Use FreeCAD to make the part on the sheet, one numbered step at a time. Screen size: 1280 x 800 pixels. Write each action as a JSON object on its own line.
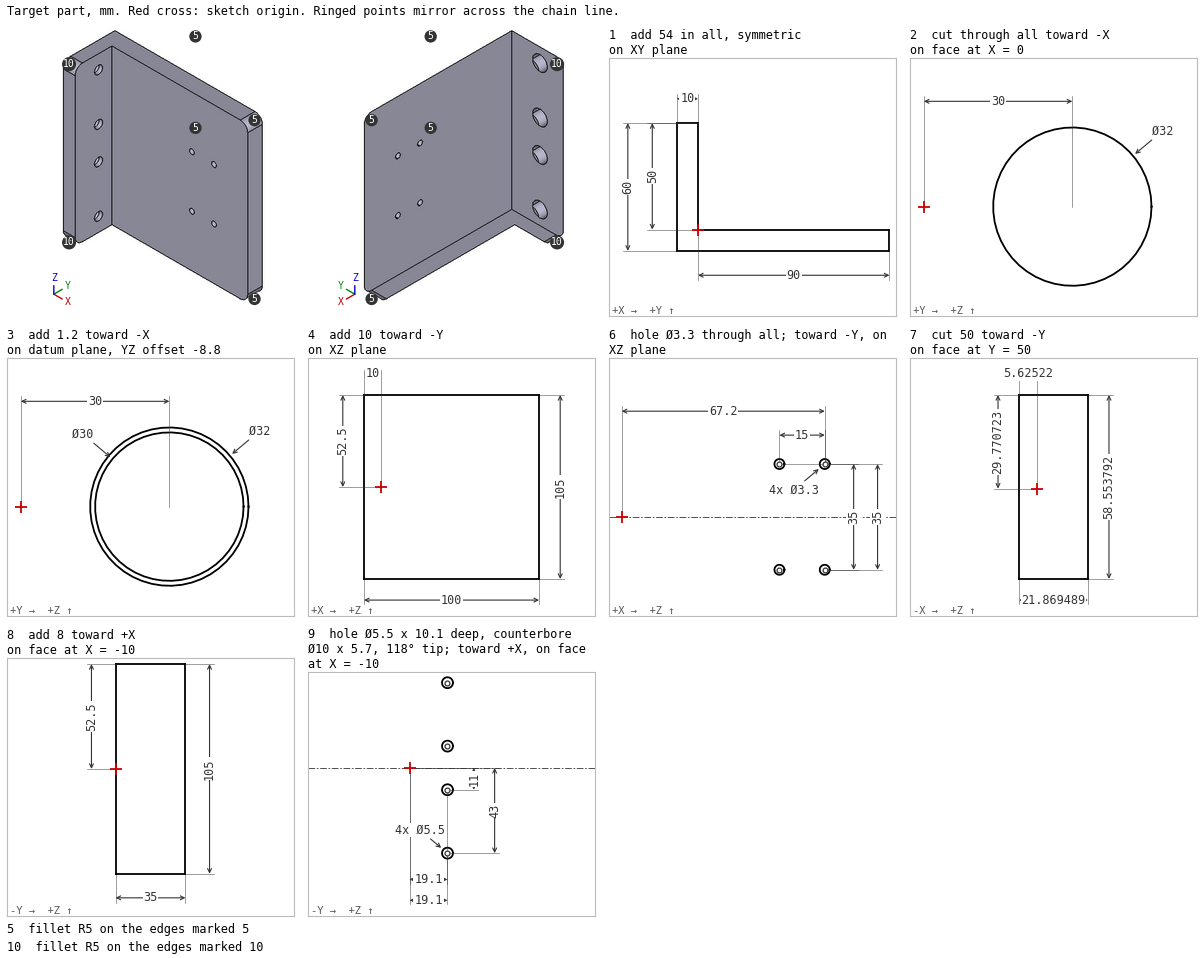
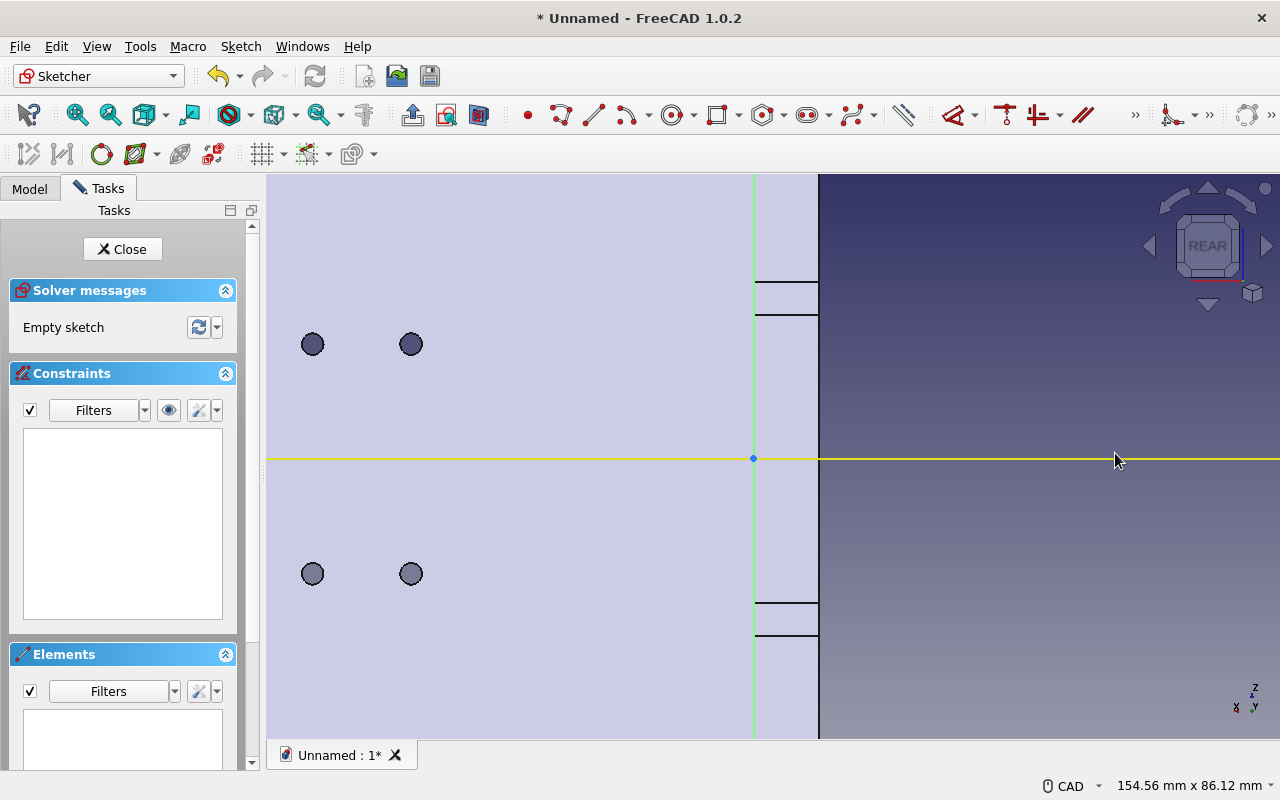
{"action": "left_click", "coordinate": [716, 116]}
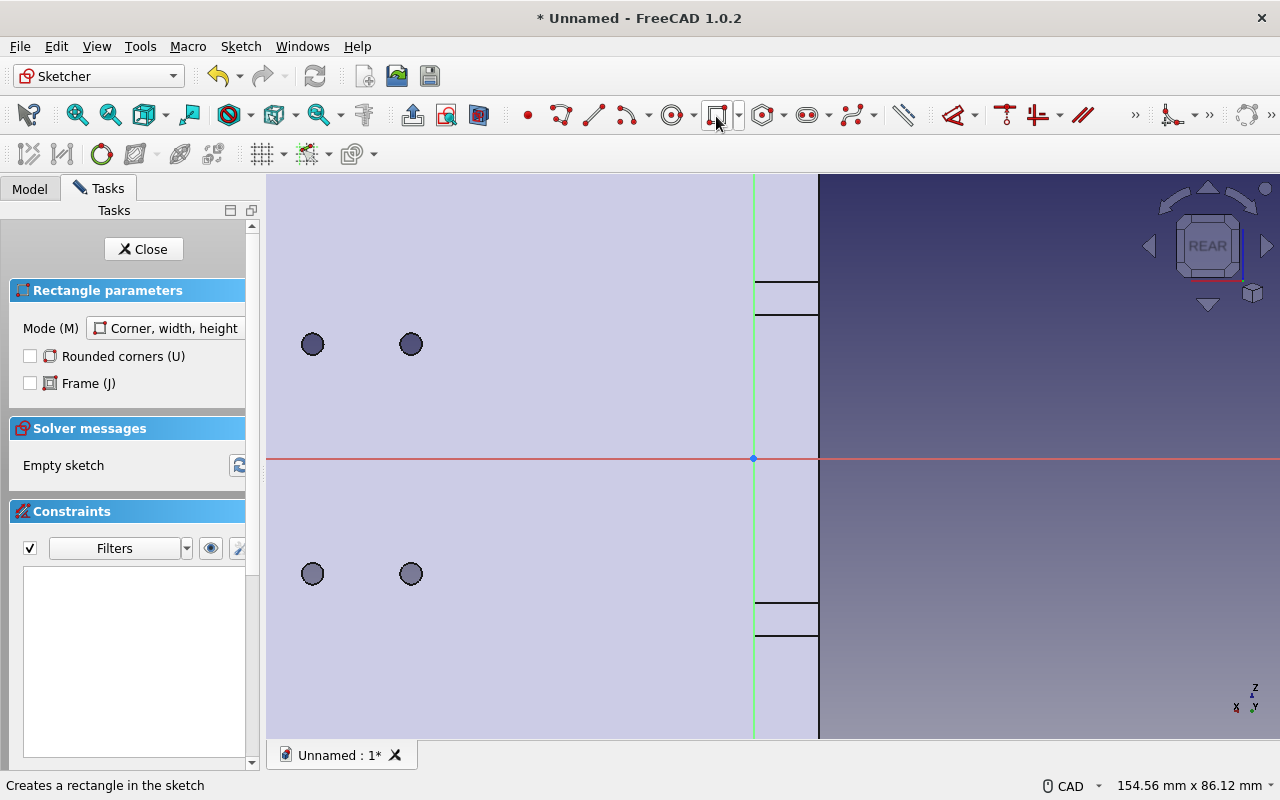
{"action": "left_click", "coordinate": [717, 264]}
{"action": "mouse_move", "coordinate": [860, 648]}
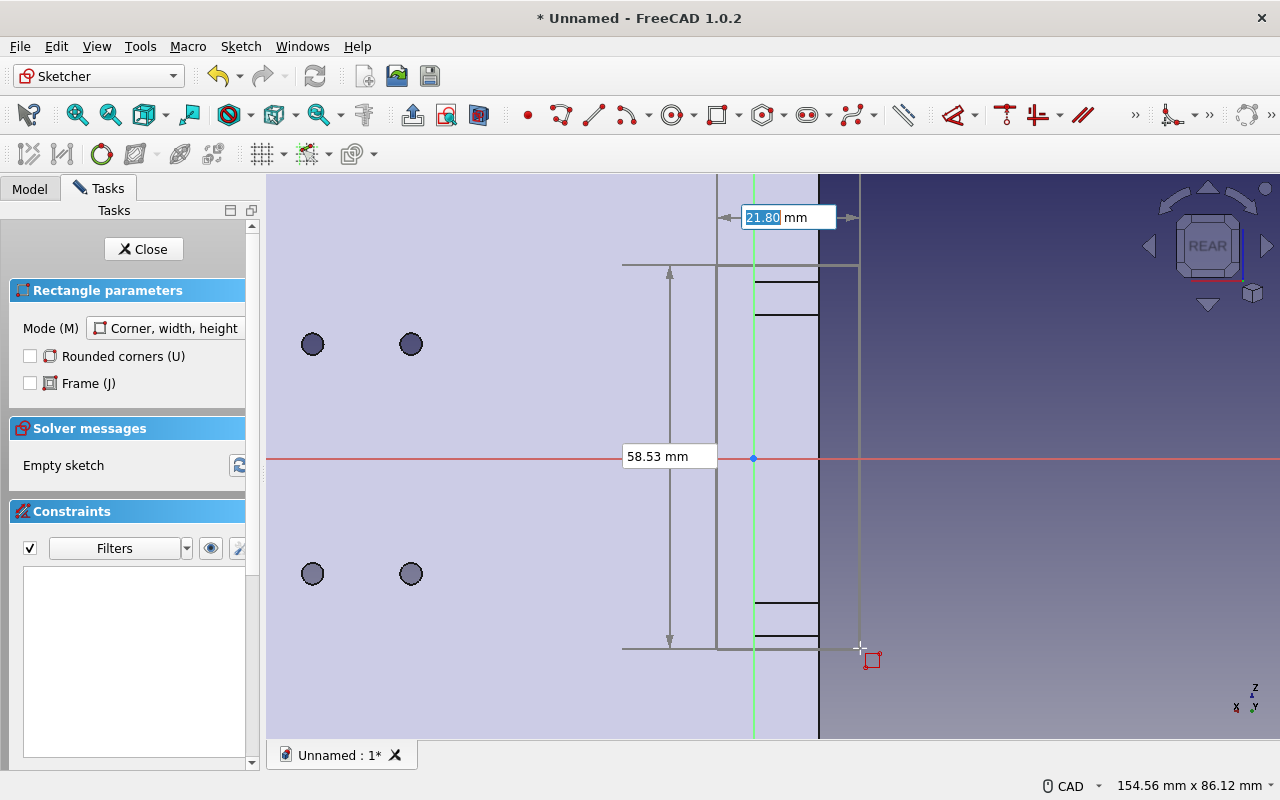
{"action": "type", "text": "21.869489"}
{"action": "key", "text": "Tab"}
{"action": "type", "text": "58.553792"}
{"action": "key", "text": "Return"}
{"action": "key", "text": "Escape"}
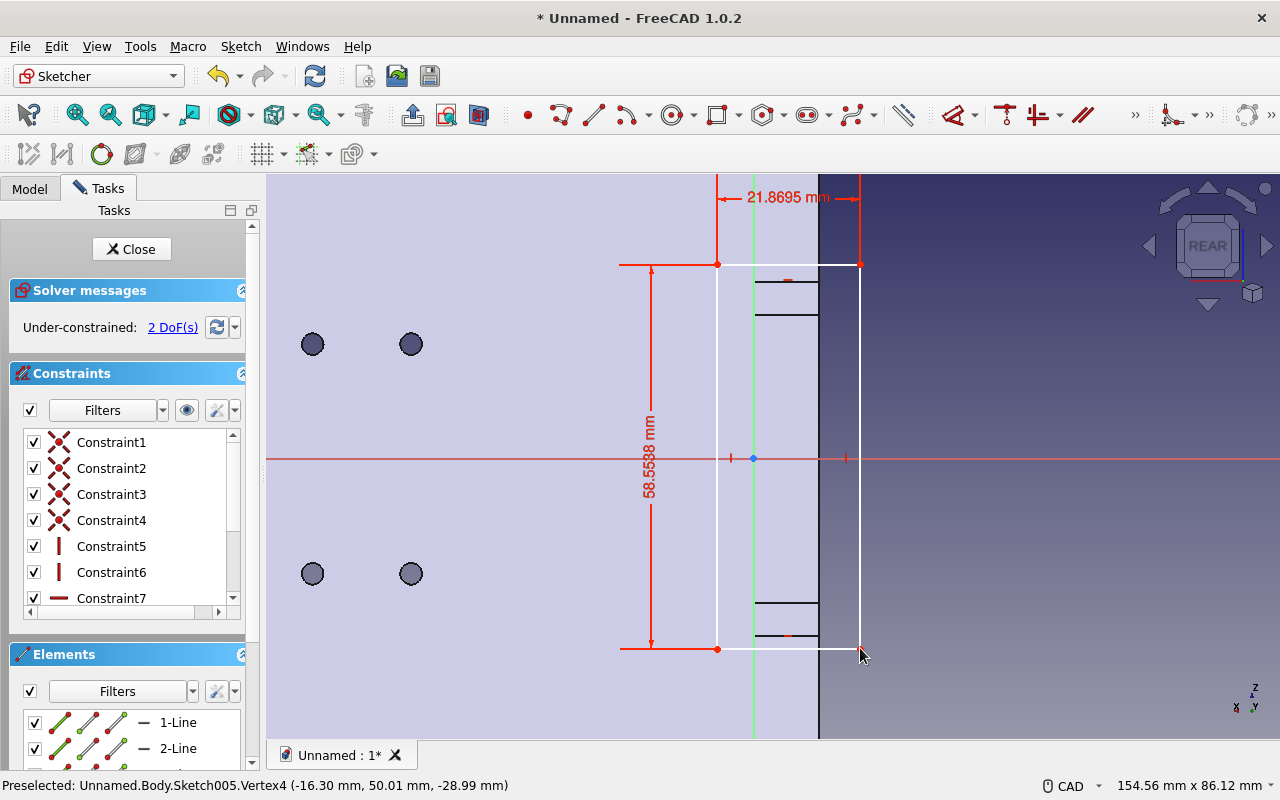
{"action": "left_click", "coordinate": [952, 116]}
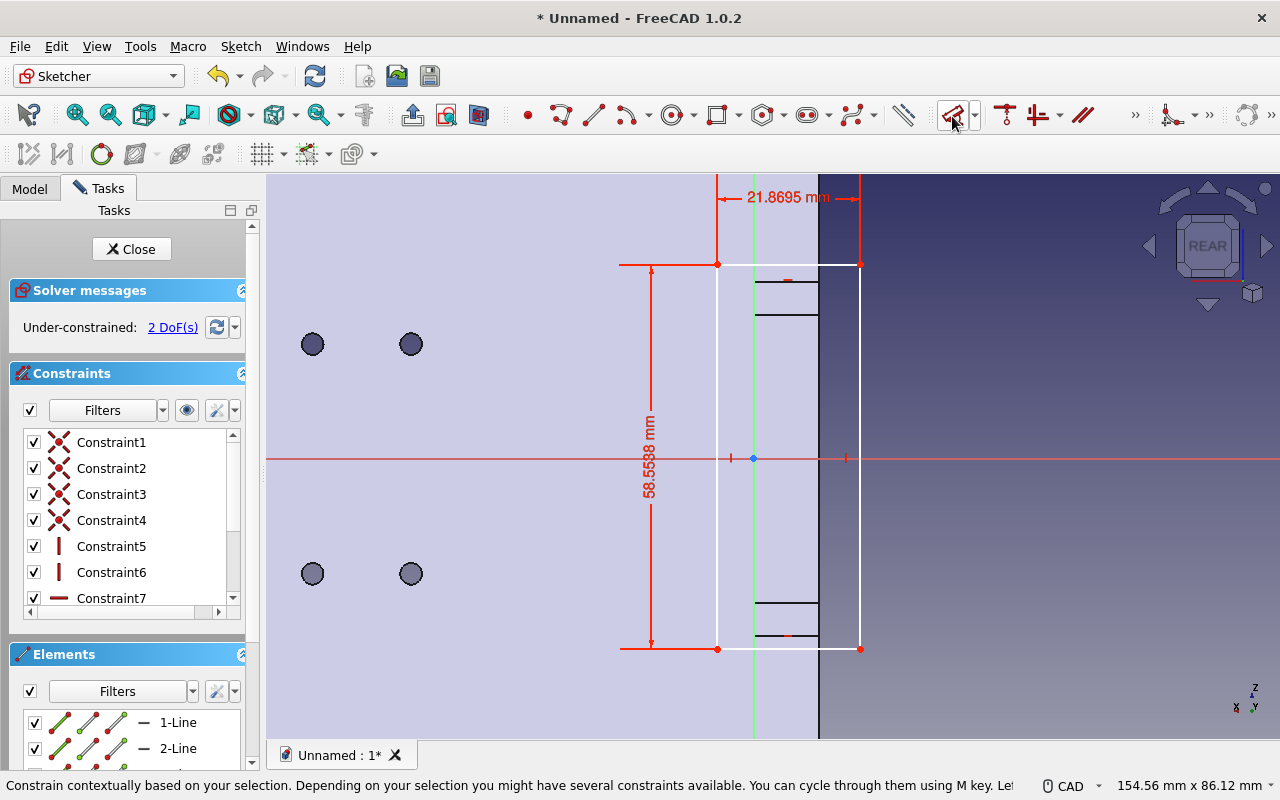
{"action": "left_click", "coordinate": [717, 265]}
{"action": "left_click", "coordinate": [735, 231]}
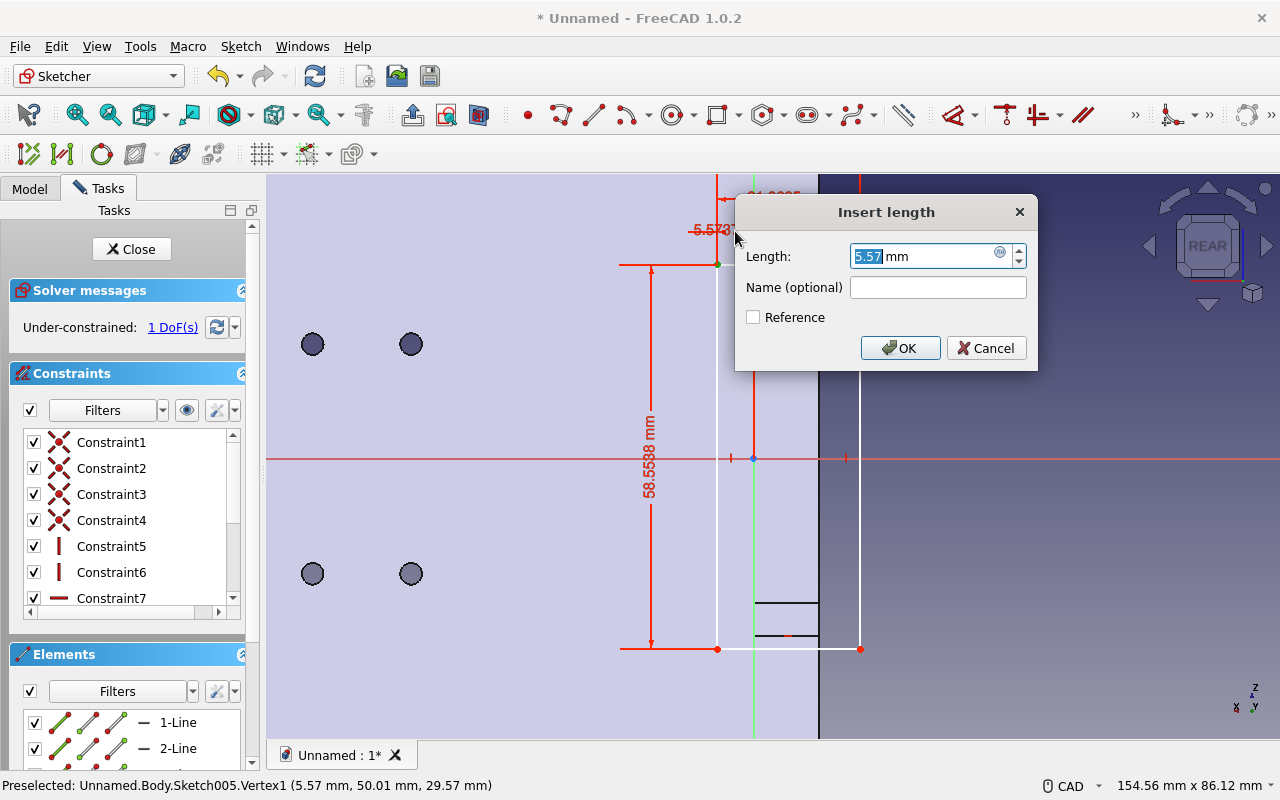
{"action": "type", "text": "5.62522"}
{"action": "key", "text": "Return"}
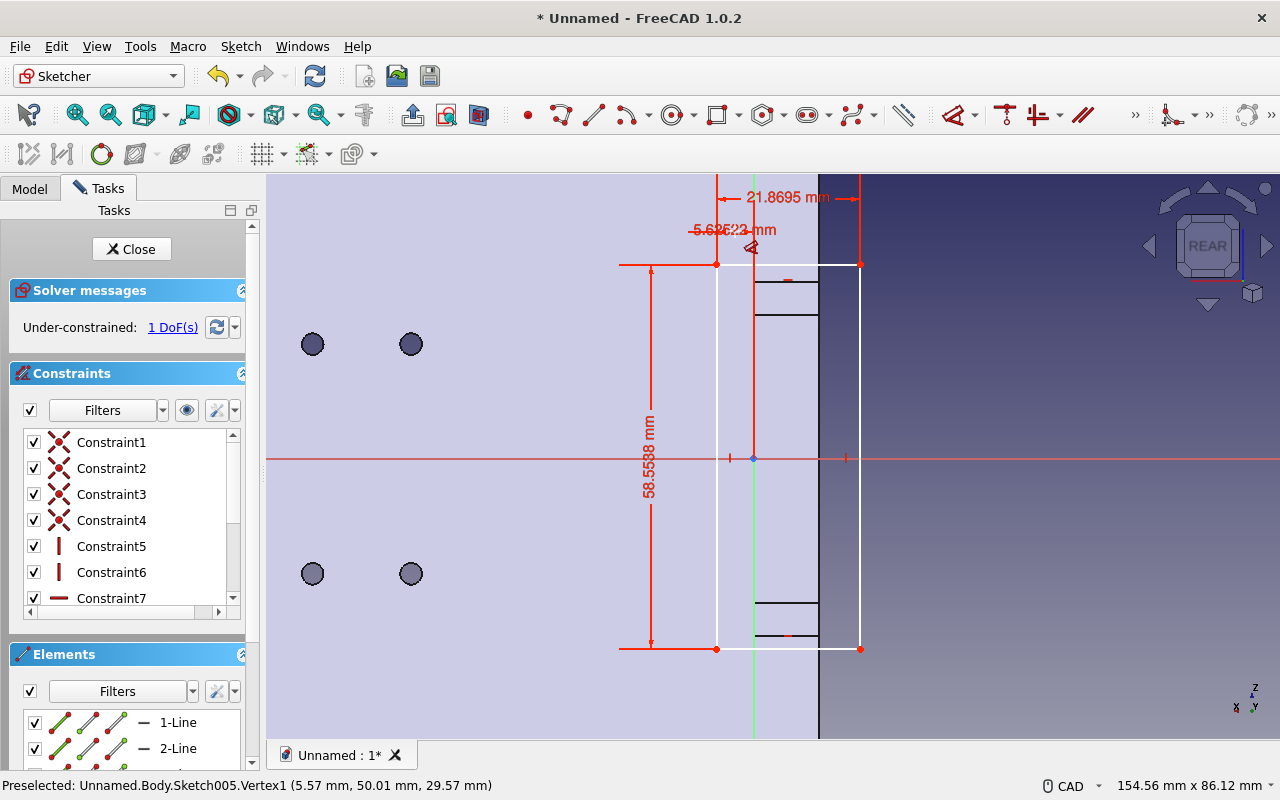
{"action": "left_click", "coordinate": [717, 265]}
{"action": "left_click", "coordinate": [683, 362]}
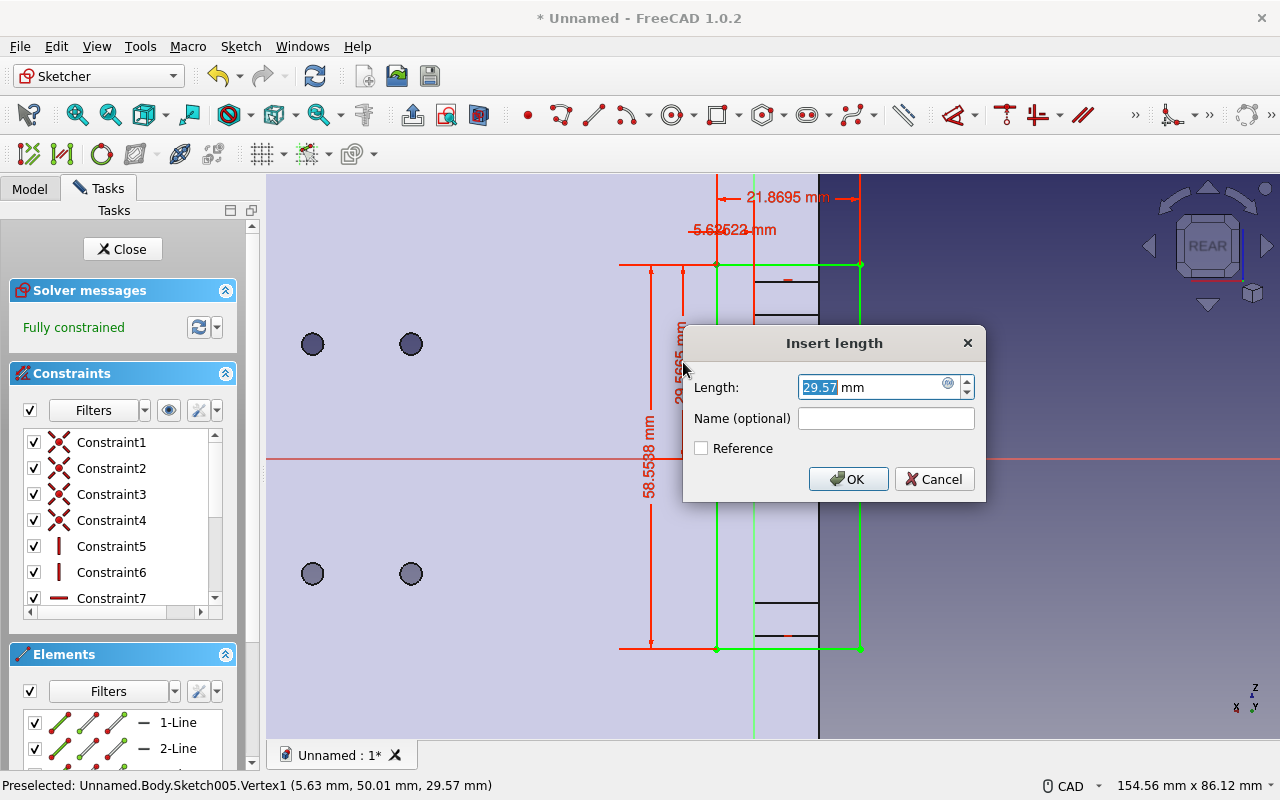
{"action": "type", "text": "29.770723"}
{"action": "key", "text": "Return"}
{"action": "key", "text": "Escape"}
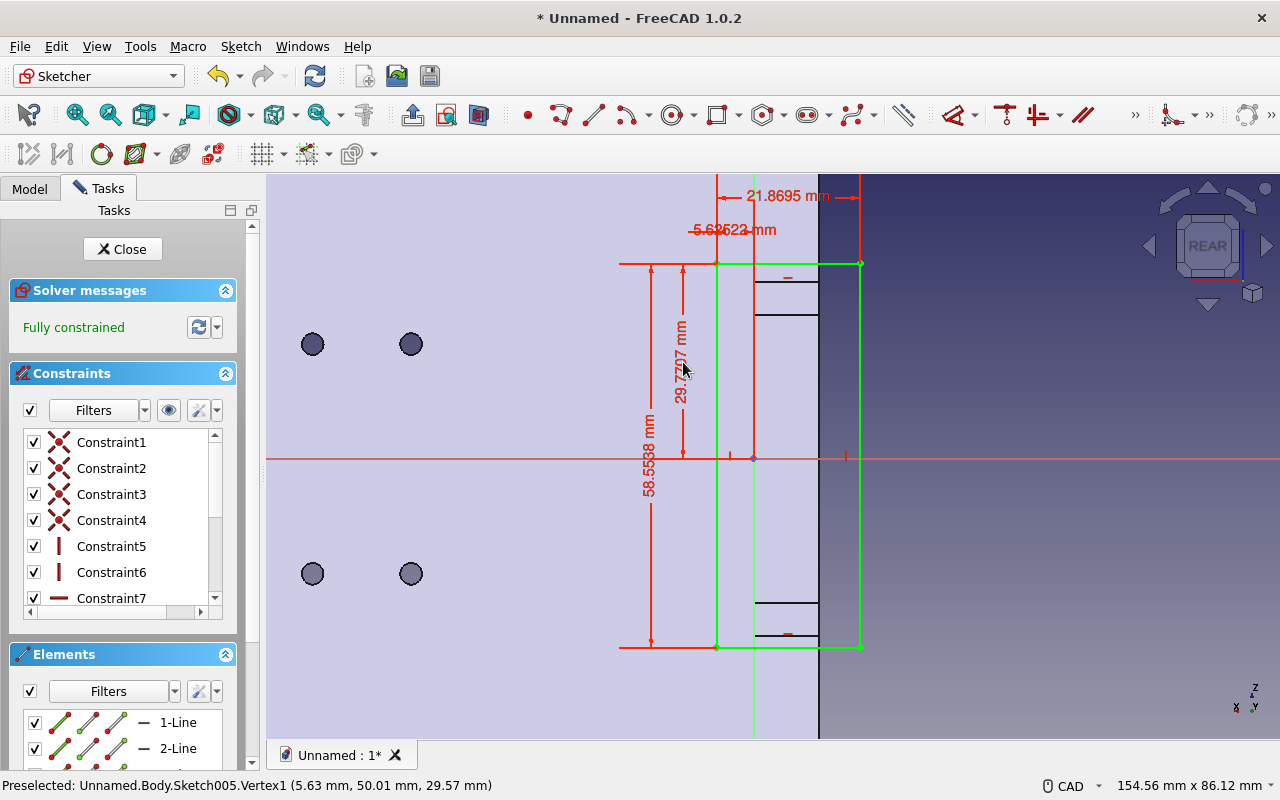
{"action": "left_click", "coordinate": [123, 249]}